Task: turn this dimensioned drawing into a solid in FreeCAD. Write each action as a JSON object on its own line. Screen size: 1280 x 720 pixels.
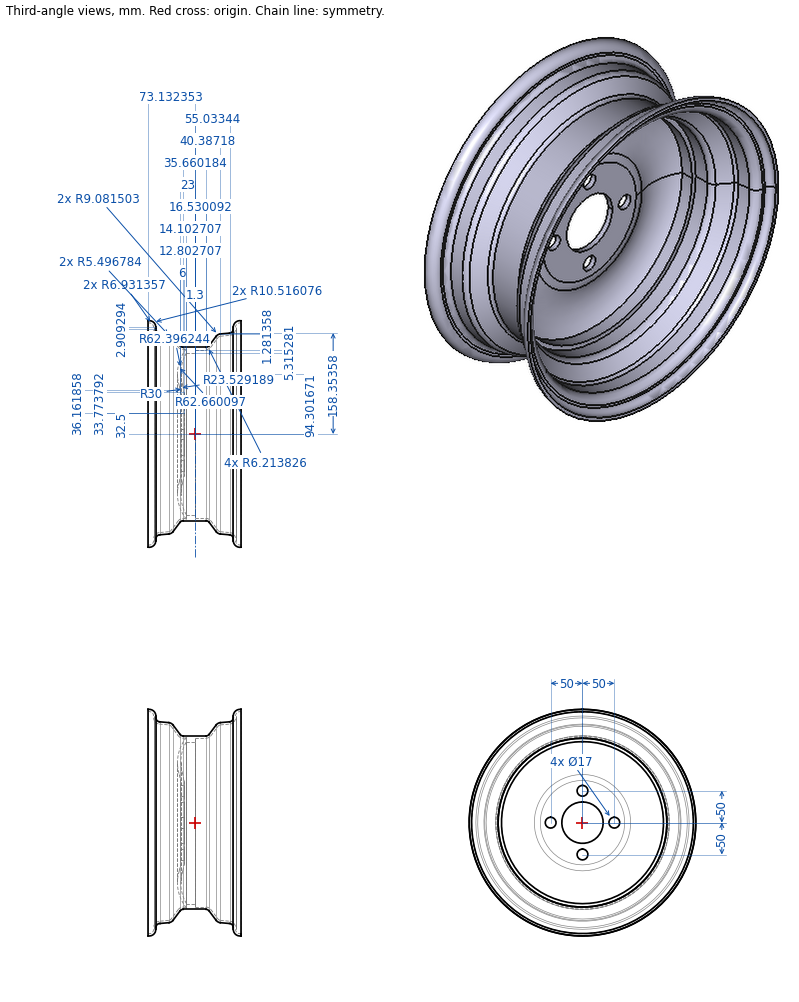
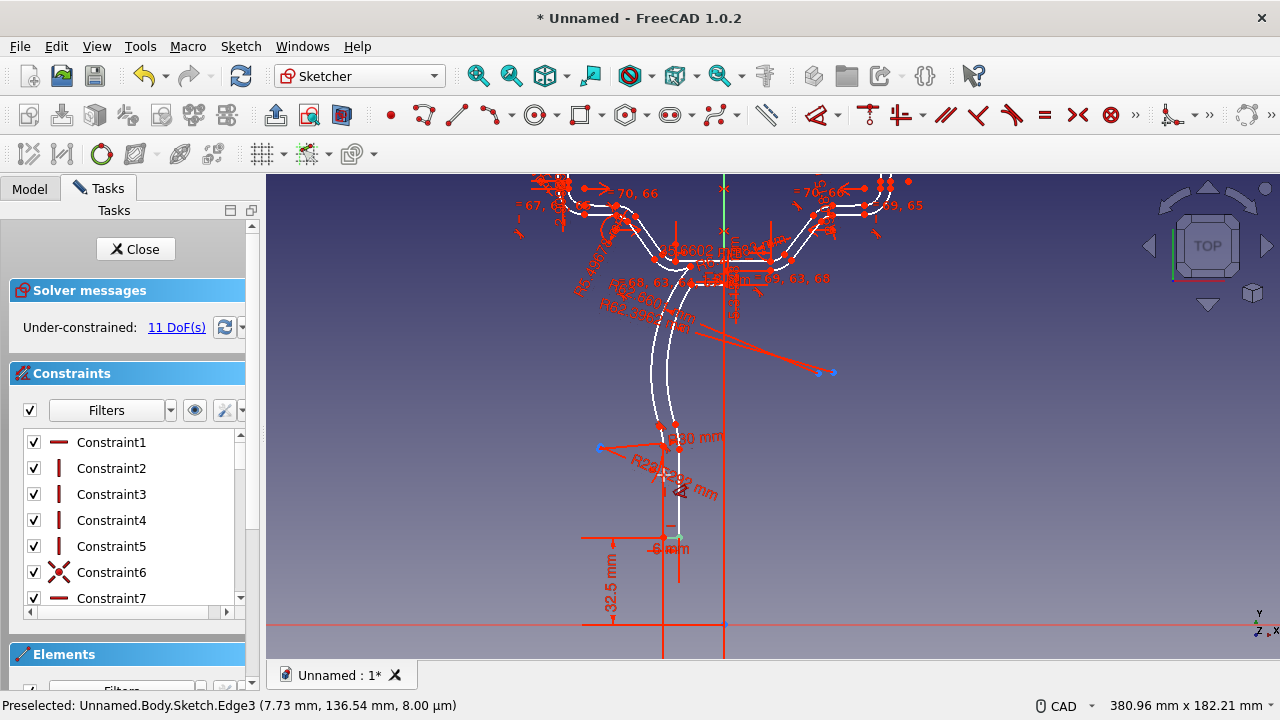
{"action": "left_click", "coordinate": [663, 474]}
{"action": "left_click", "coordinate": [629, 513]}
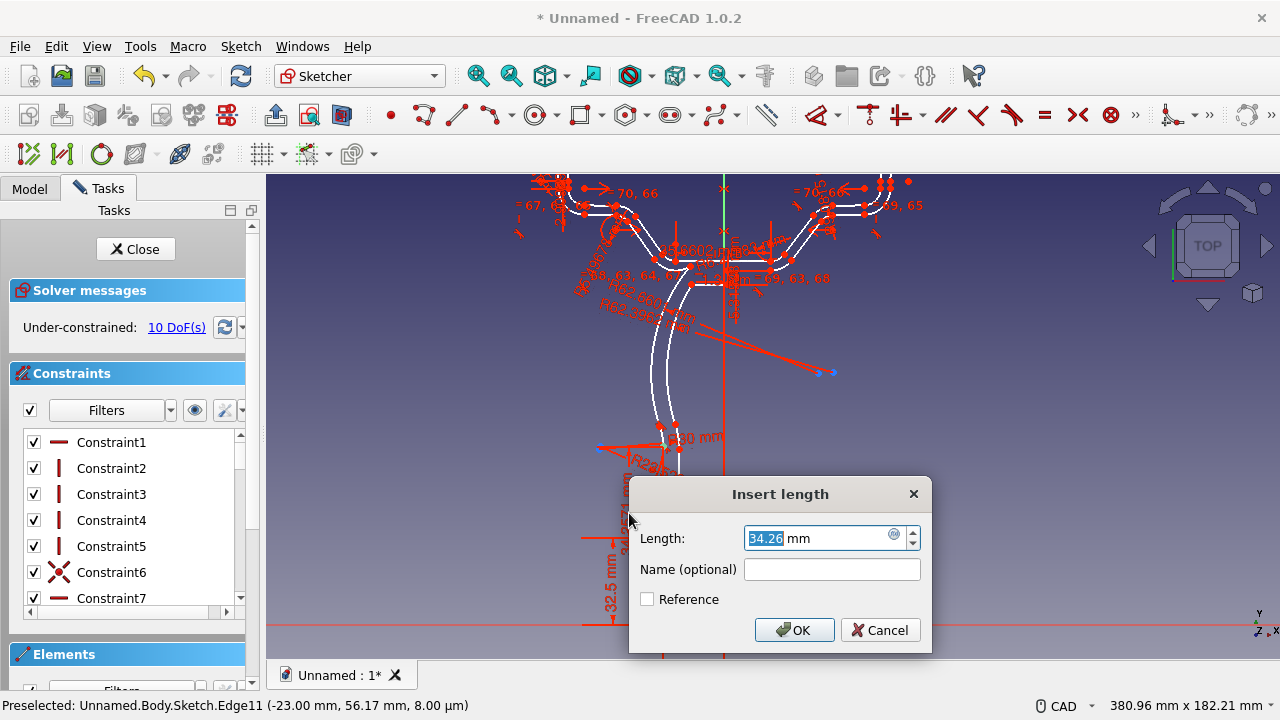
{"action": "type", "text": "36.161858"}
{"action": "key", "text": "Return"}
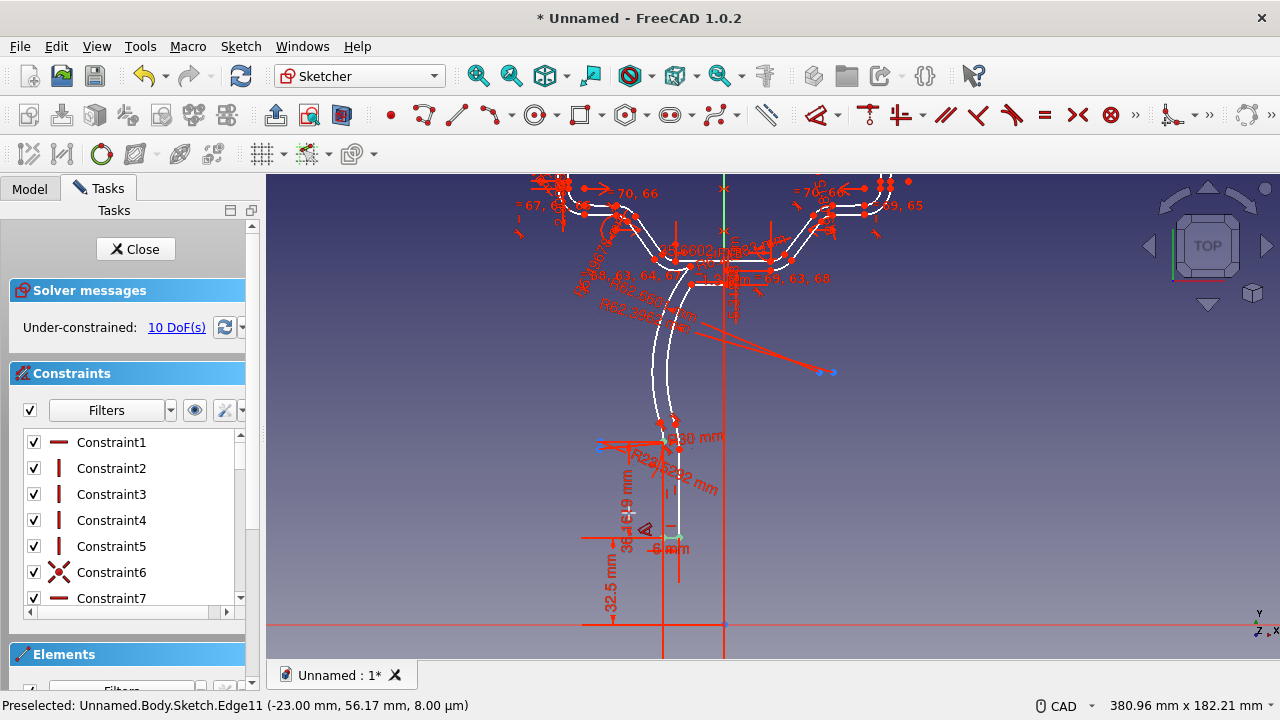
{"action": "left_click", "coordinate": [679, 511]}
{"action": "left_click", "coordinate": [645, 462]}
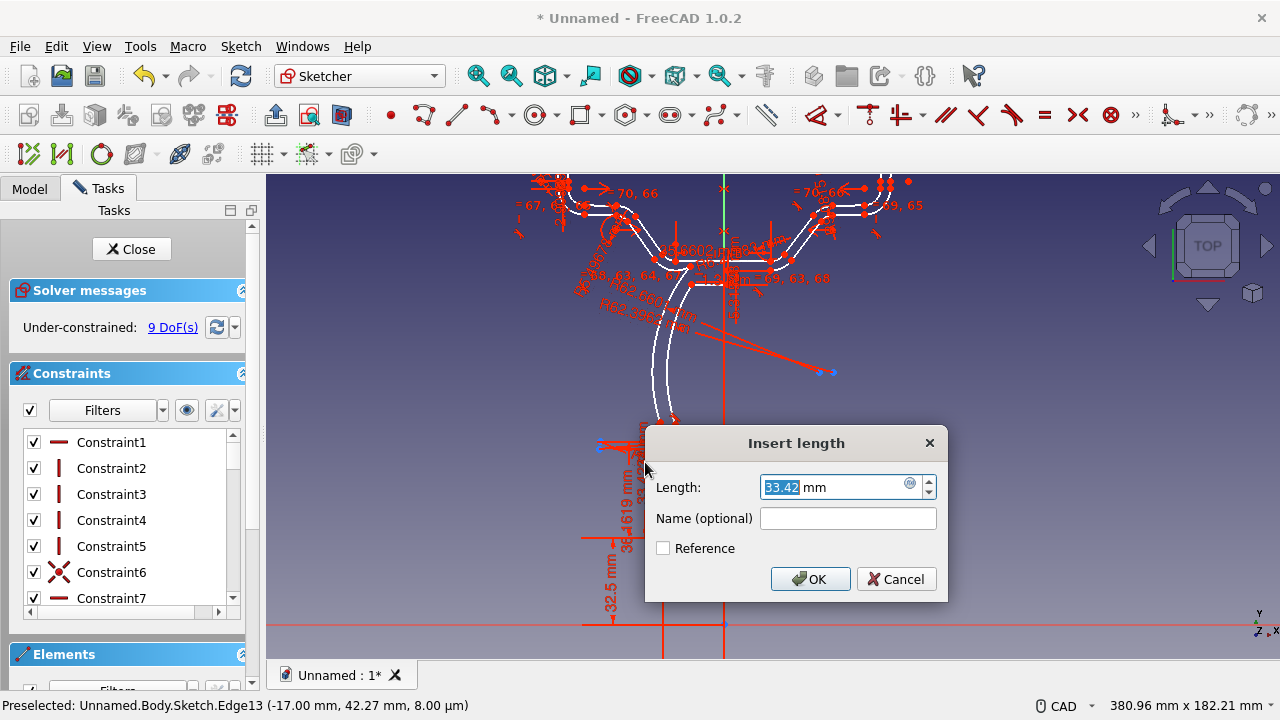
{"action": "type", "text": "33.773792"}
{"action": "key", "text": "Return"}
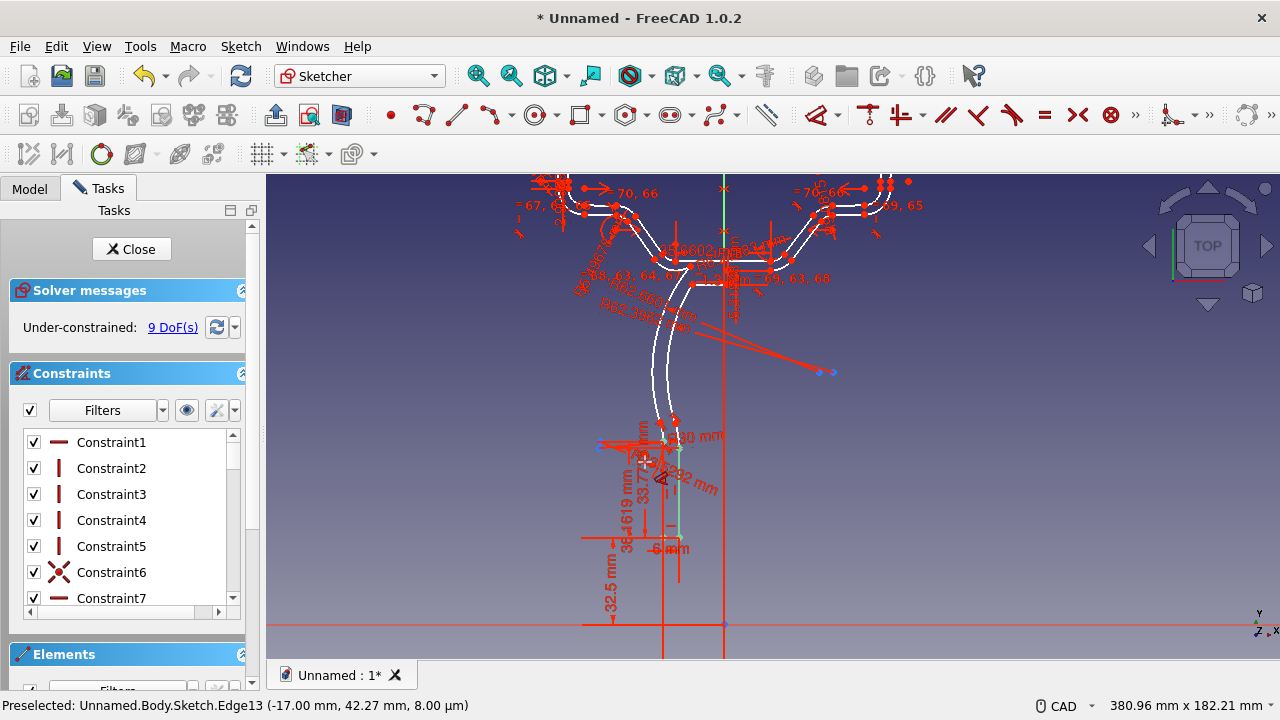
{"action": "scroll", "coordinate": [703, 285], "scroll_direction": "up", "scroll_amount": 2}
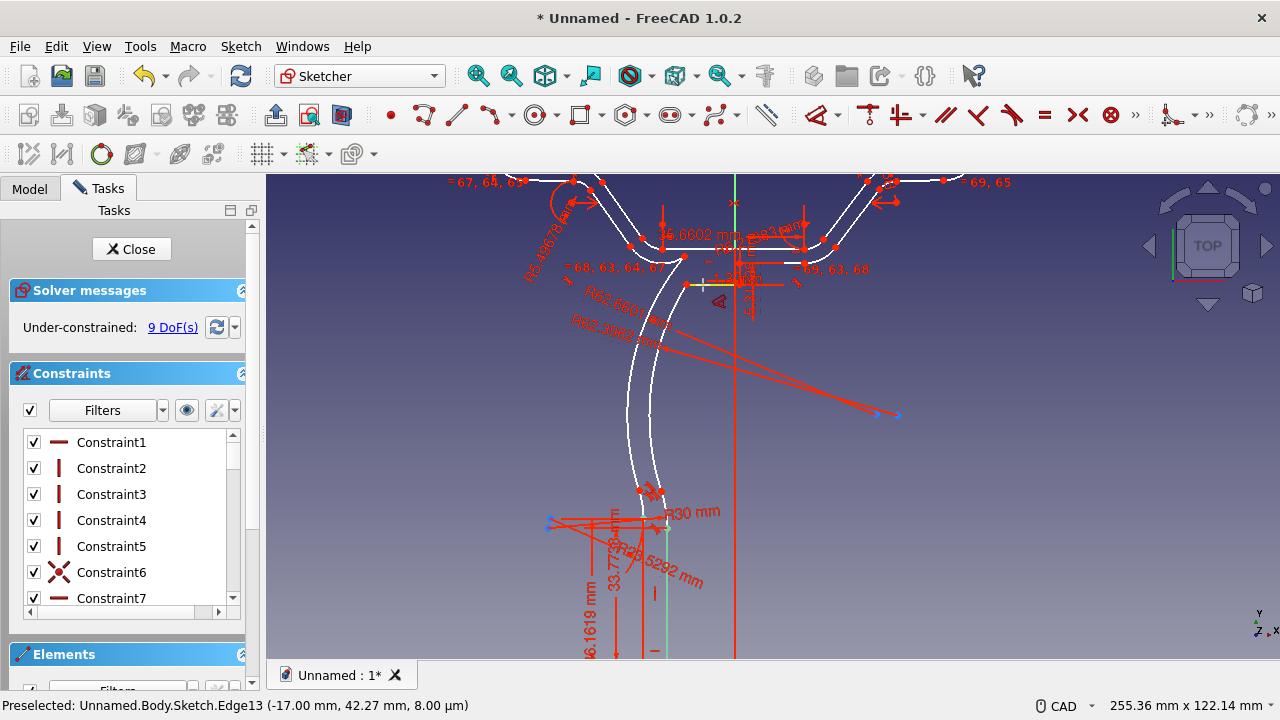
{"action": "left_click", "coordinate": [703, 285]}
{"action": "left_click", "coordinate": [713, 319]}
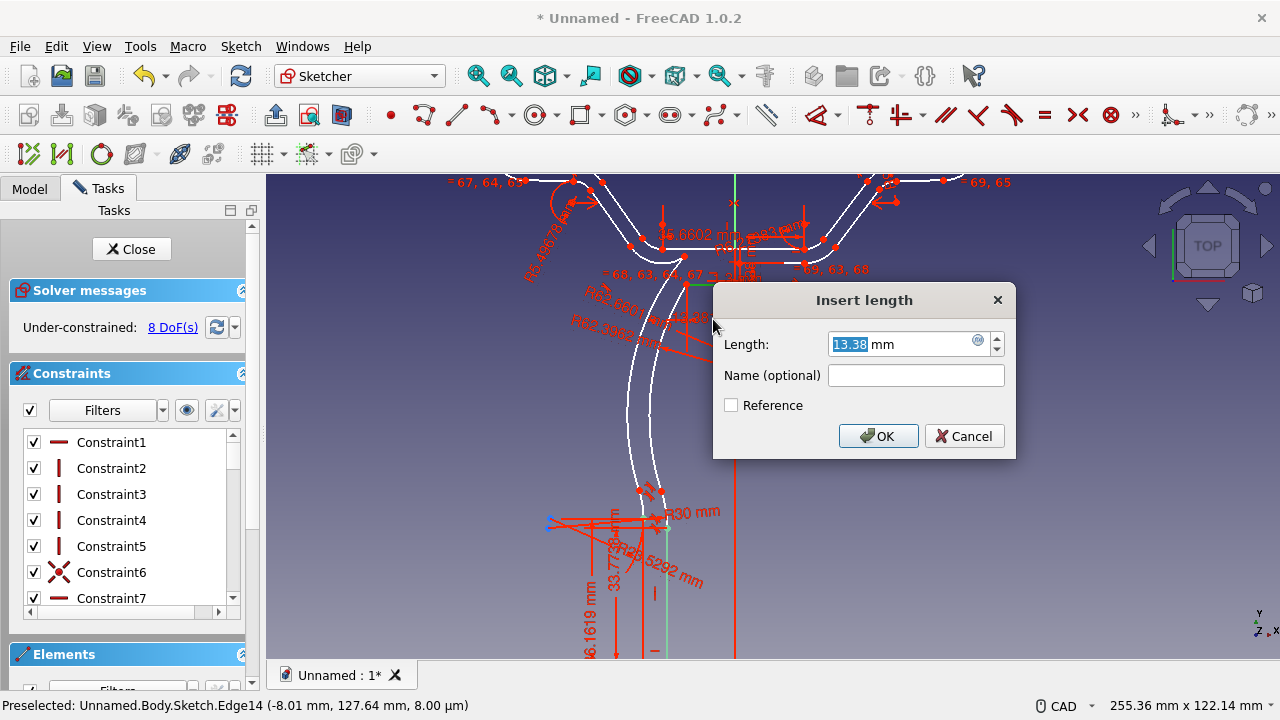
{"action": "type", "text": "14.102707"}
{"action": "key", "text": "Return"}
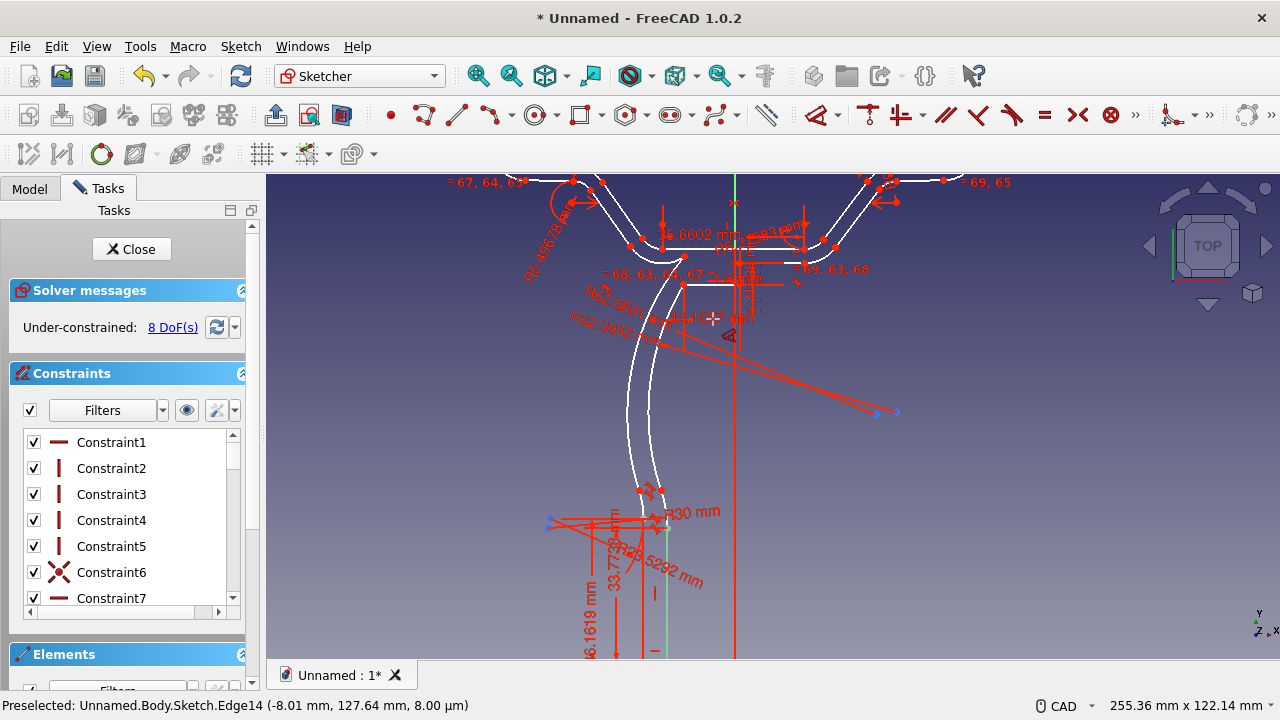
{"action": "left_click", "coordinate": [759, 263]}
{"action": "left_click", "coordinate": [787, 321]}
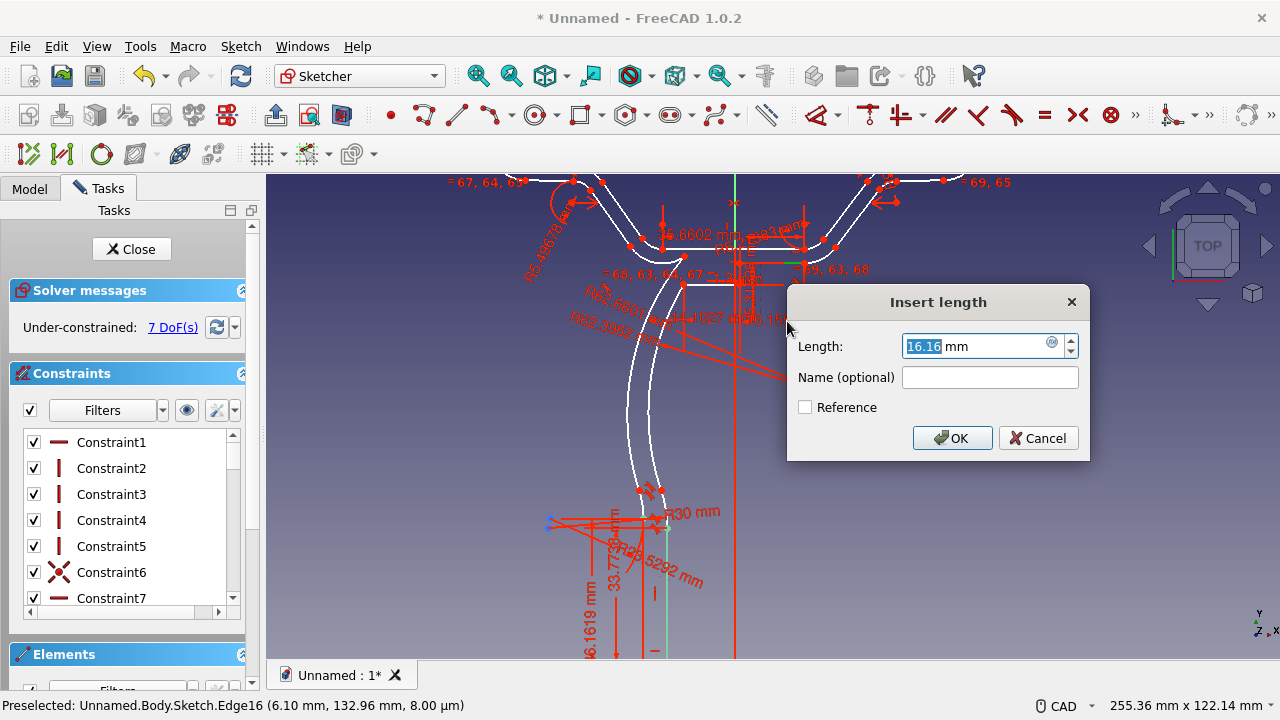
{"action": "type", "text": "16.530092"}
{"action": "key", "text": "Return"}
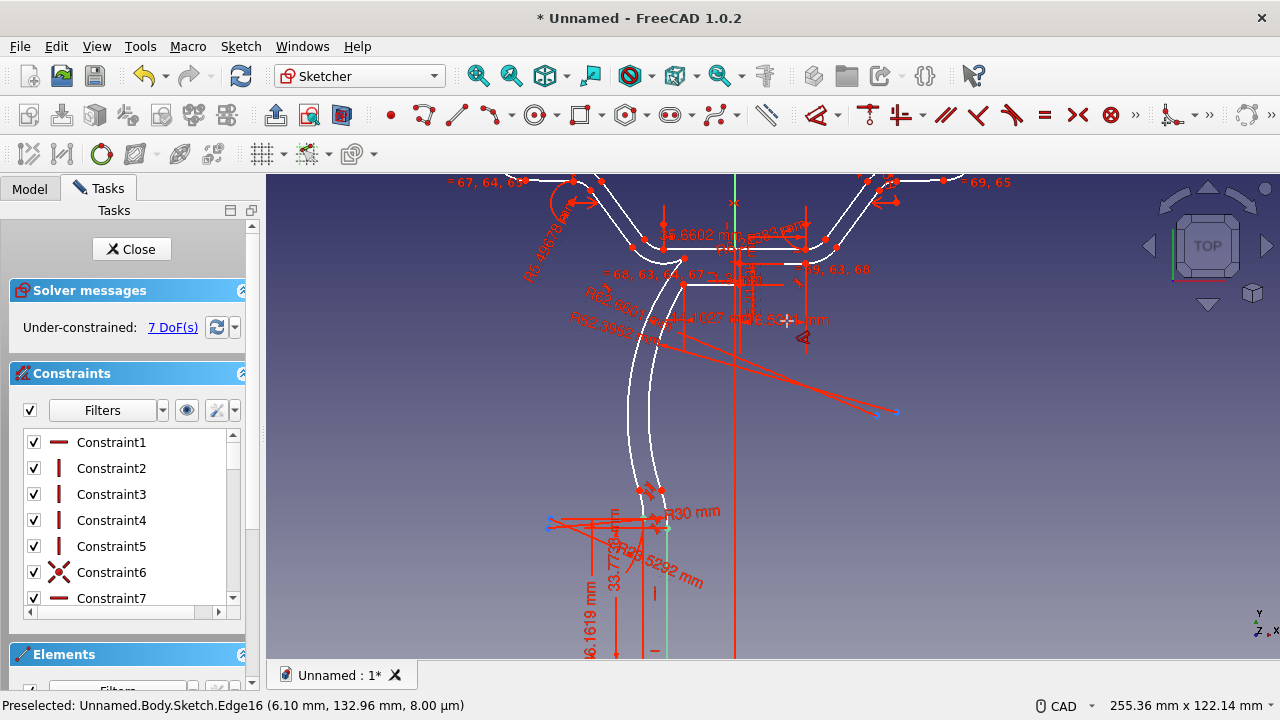
{"action": "scroll", "coordinate": [680, 399], "scroll_direction": "down", "scroll_amount": 4}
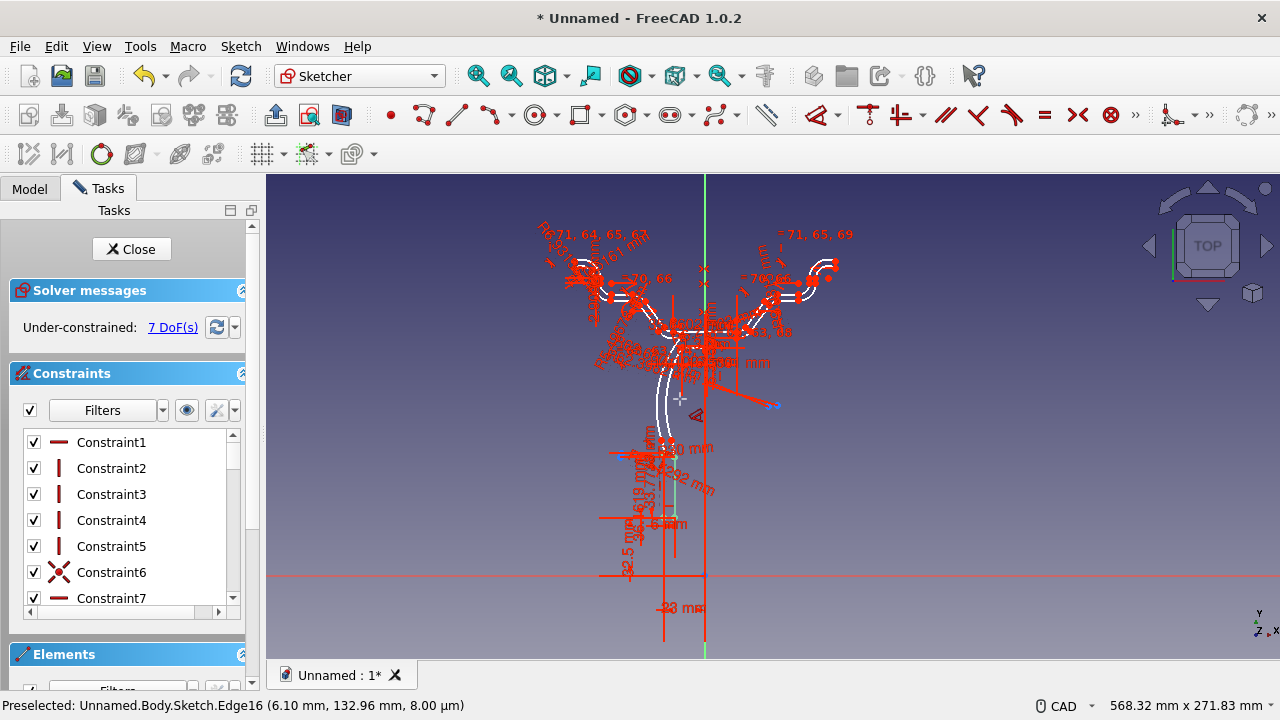
{"action": "scroll", "coordinate": [799, 295], "scroll_direction": "up", "scroll_amount": 4}